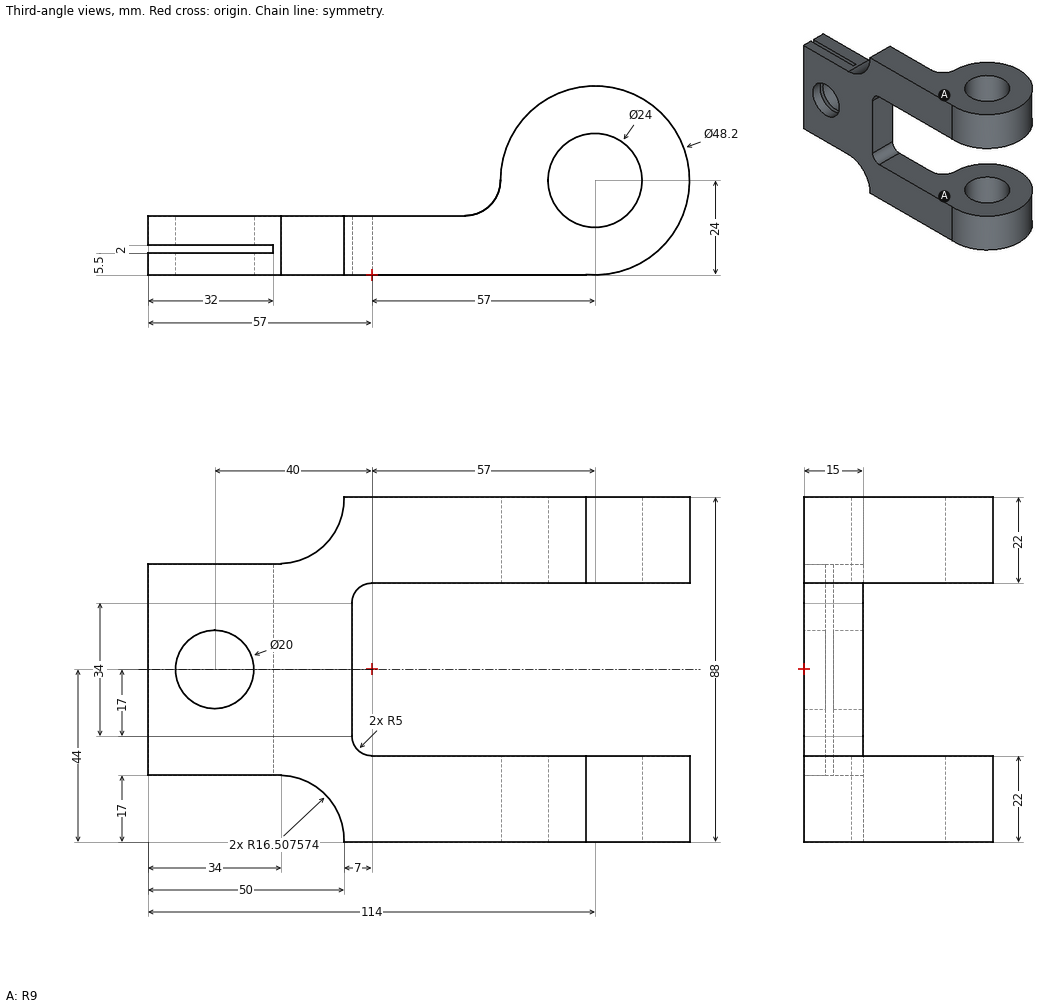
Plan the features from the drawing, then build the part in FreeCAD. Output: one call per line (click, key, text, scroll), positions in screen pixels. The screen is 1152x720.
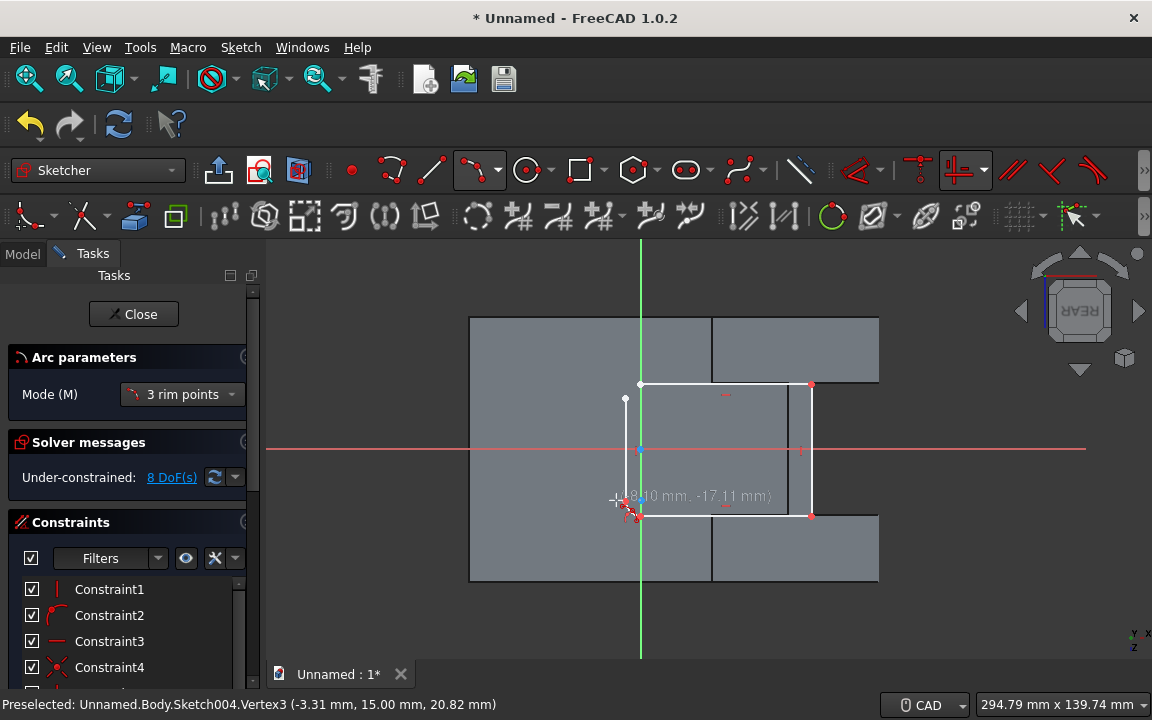
click(641, 384)
click(626, 399)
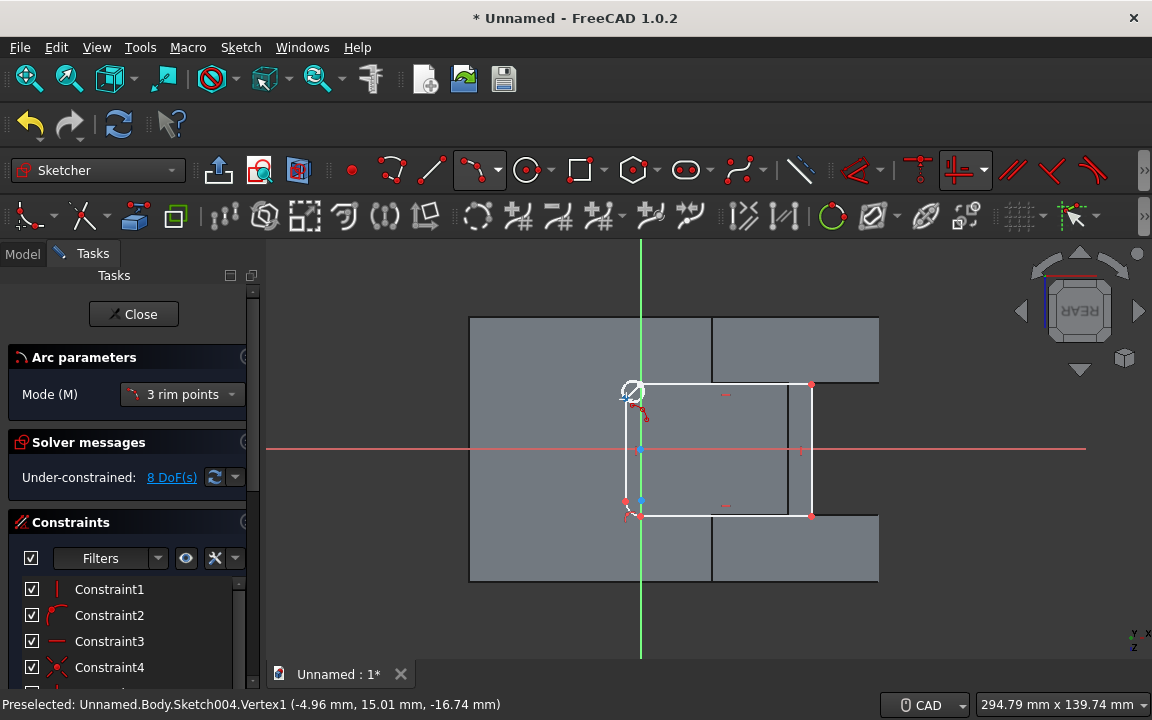
scroll(630, 388, up, 7)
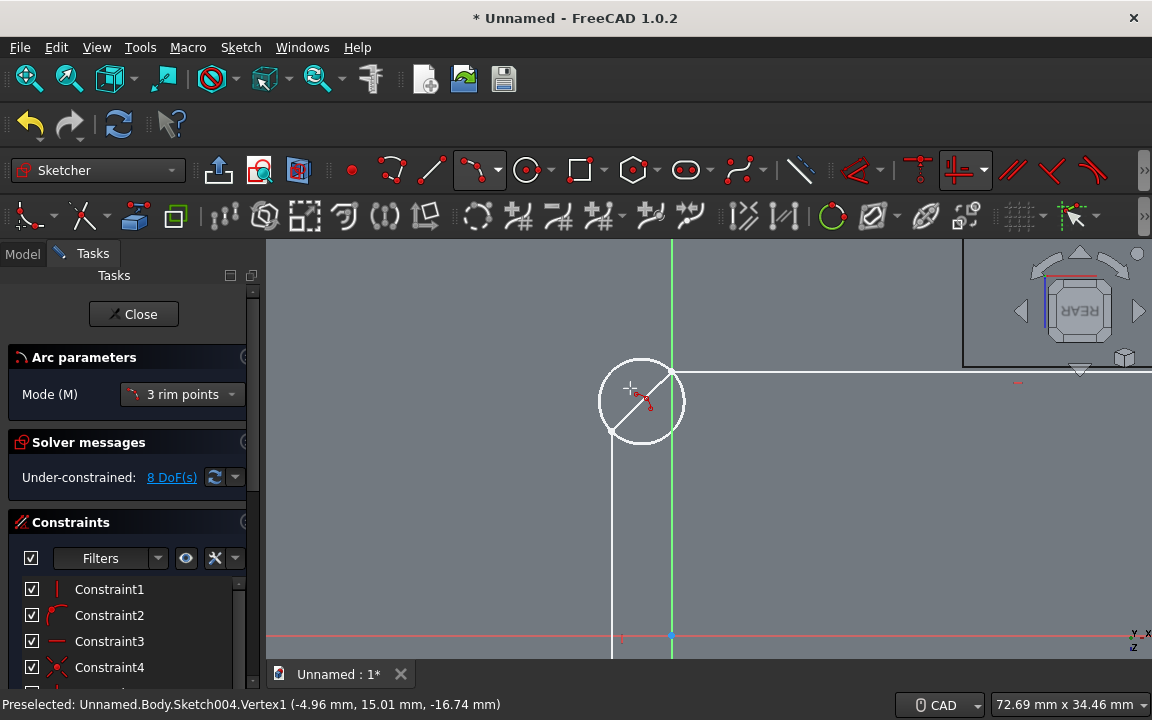
click(629, 385)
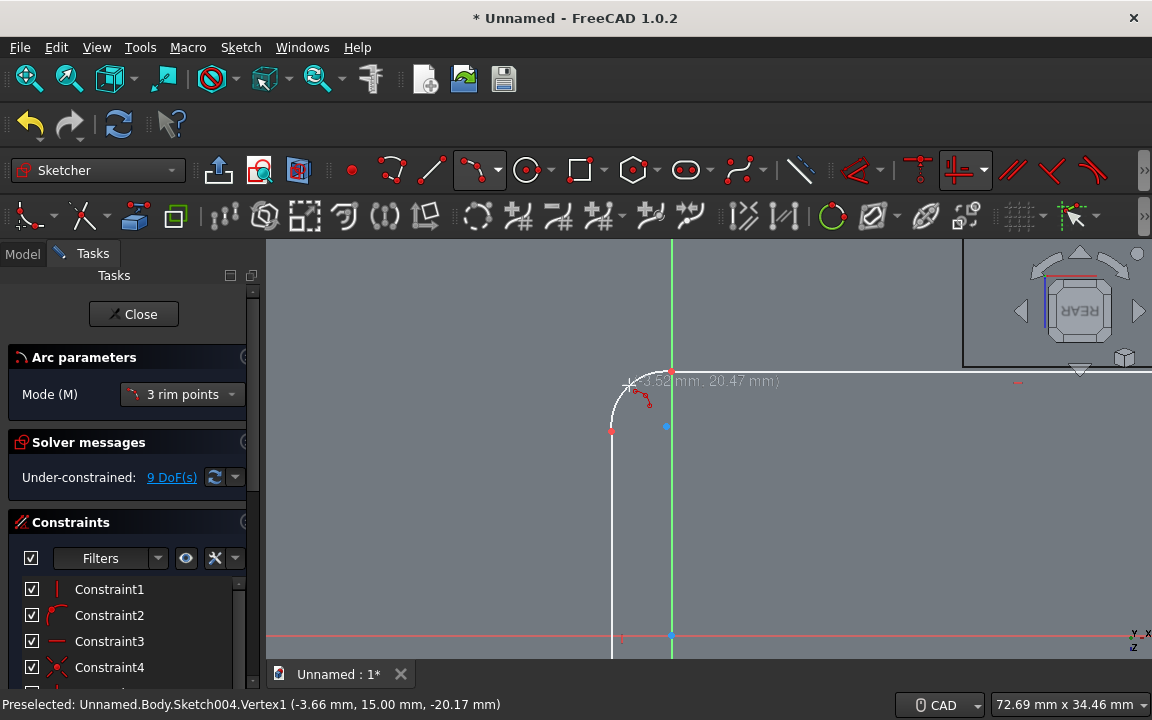
click(392, 170)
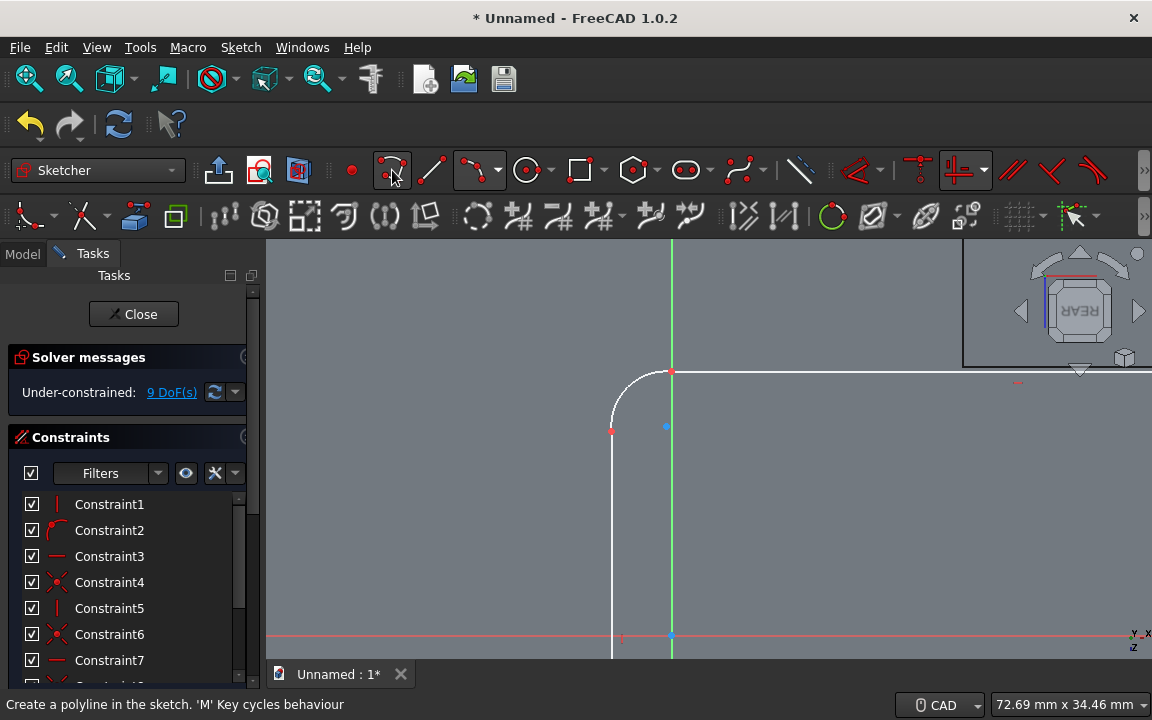
scroll(630, 388, down, 7)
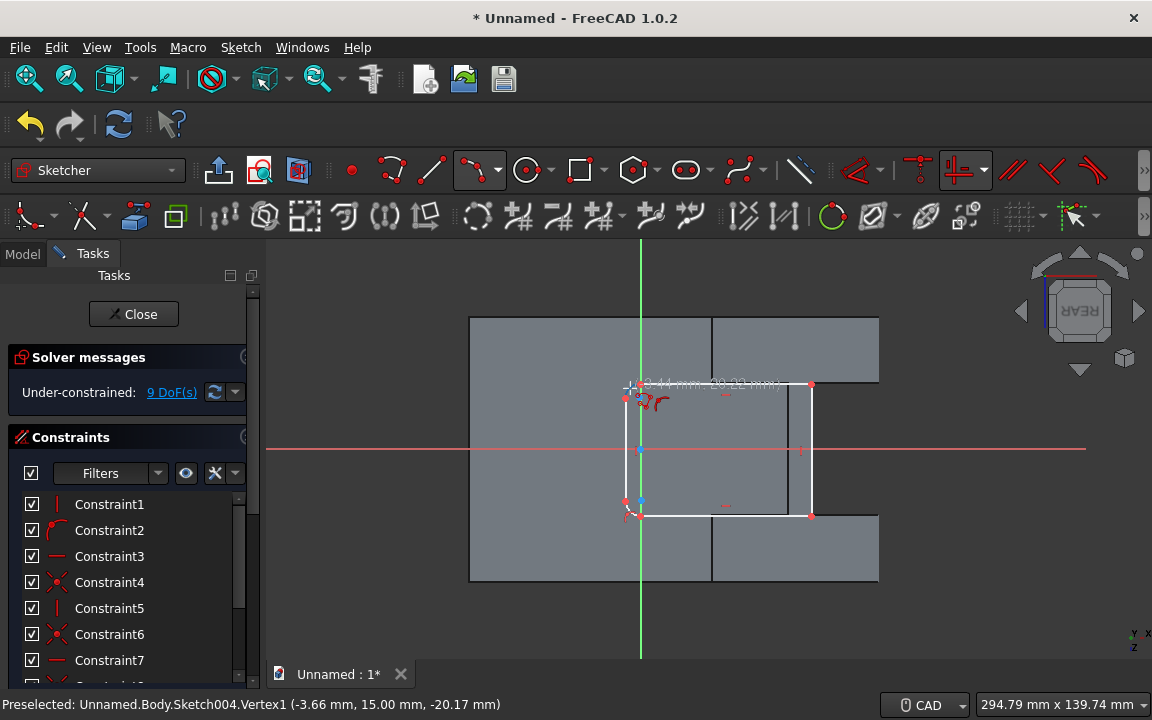
click(620, 317)
click(469, 317)
click(469, 368)
click(572, 368)
right_click(572, 368)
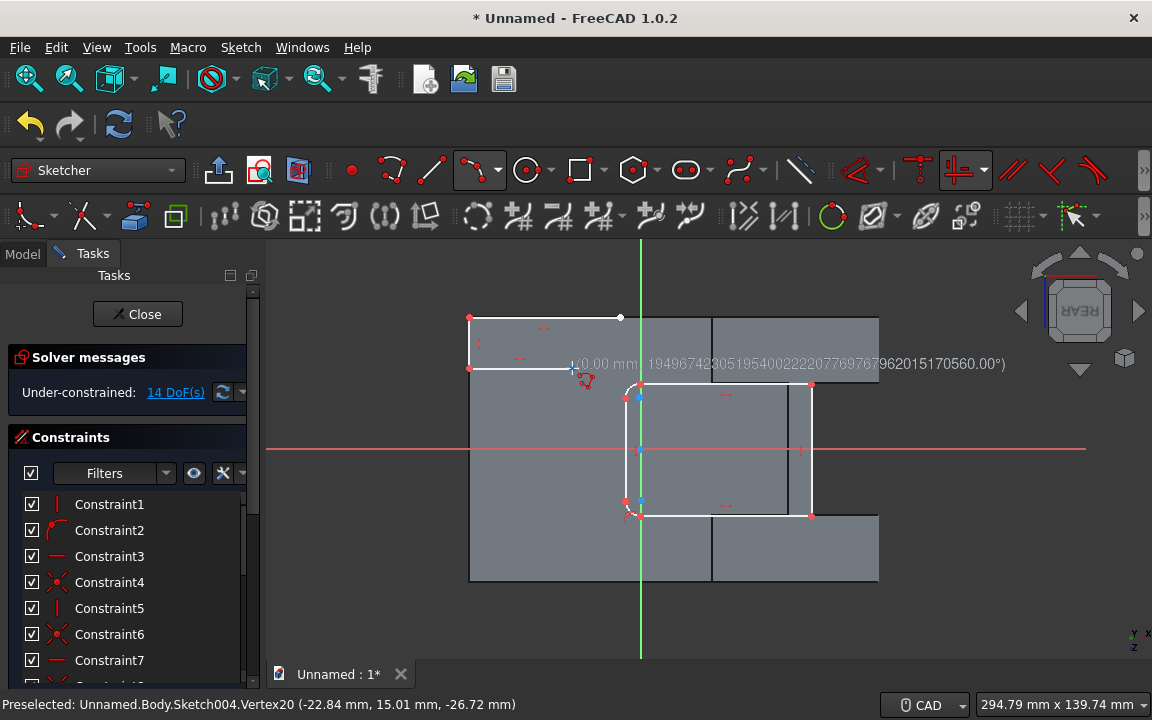
key(g)
key(3)
key(a)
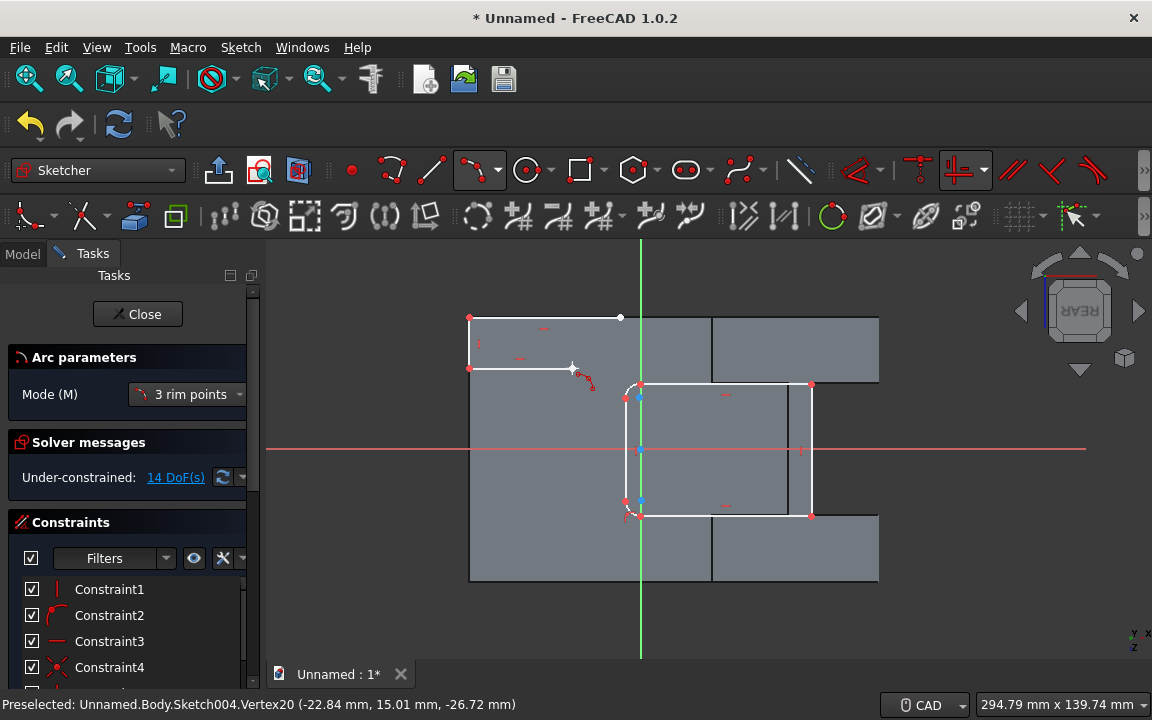
click(572, 369)
click(620, 318)
click(606, 353)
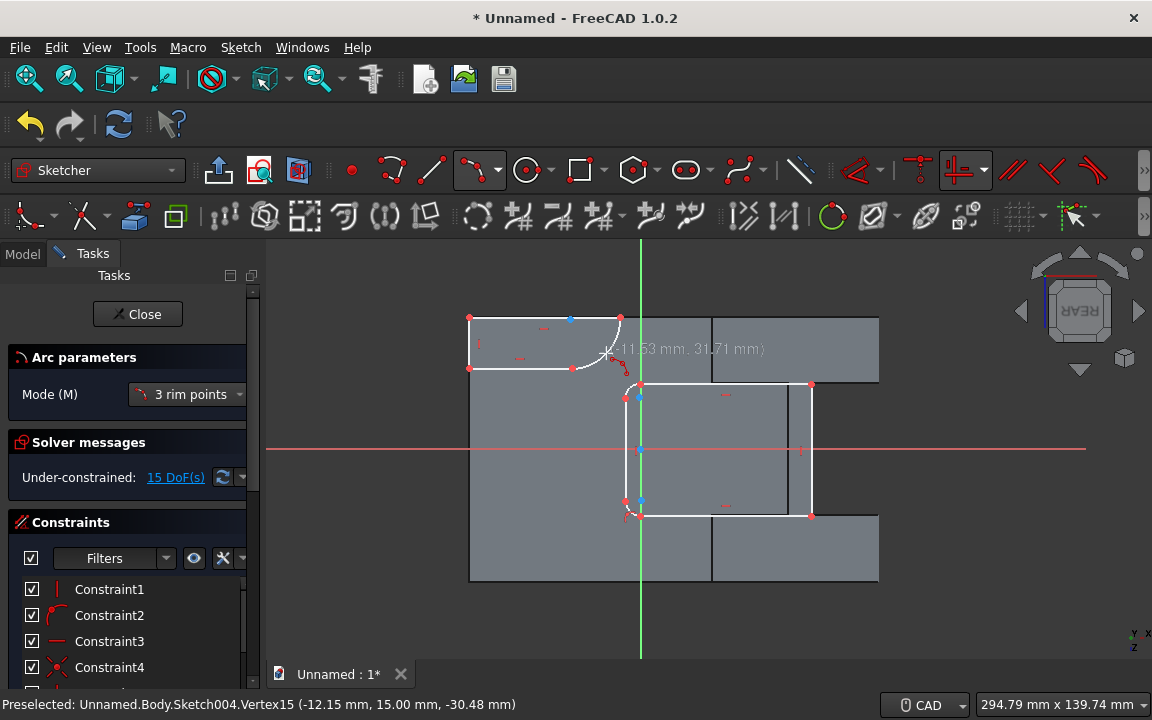
click(392, 170)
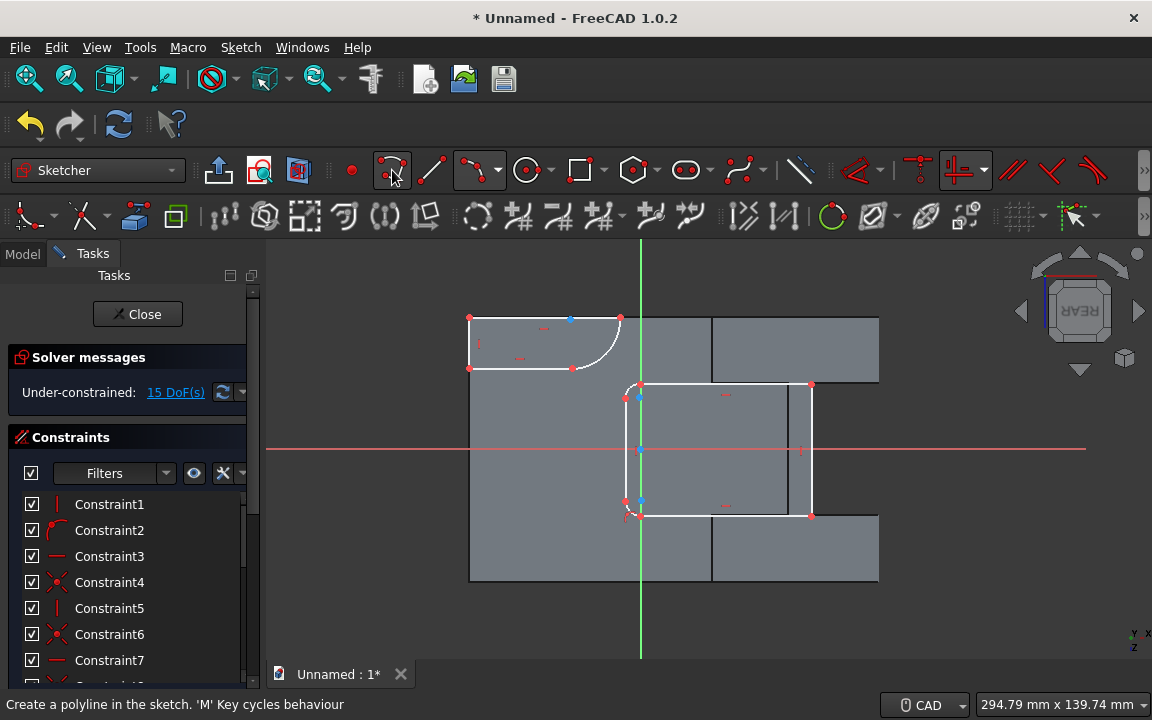
click(572, 530)
click(469, 530)
click(469, 582)
click(620, 582)
right_click(620, 582)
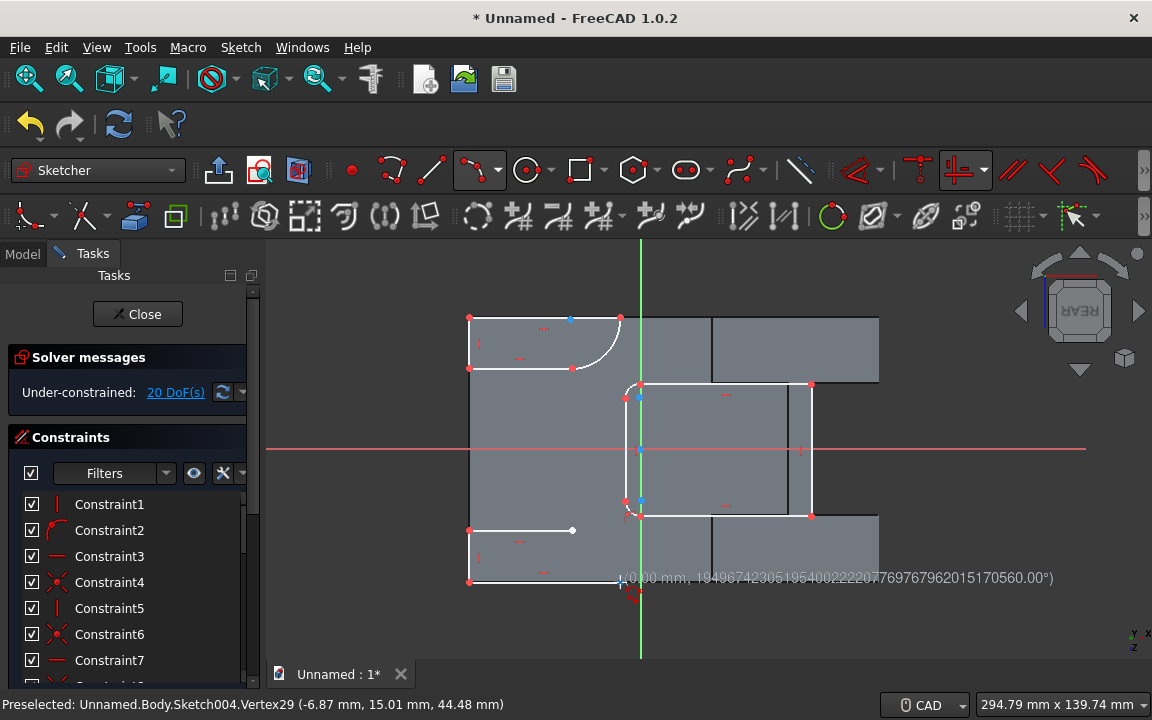
key(g)
key(3)
key(a)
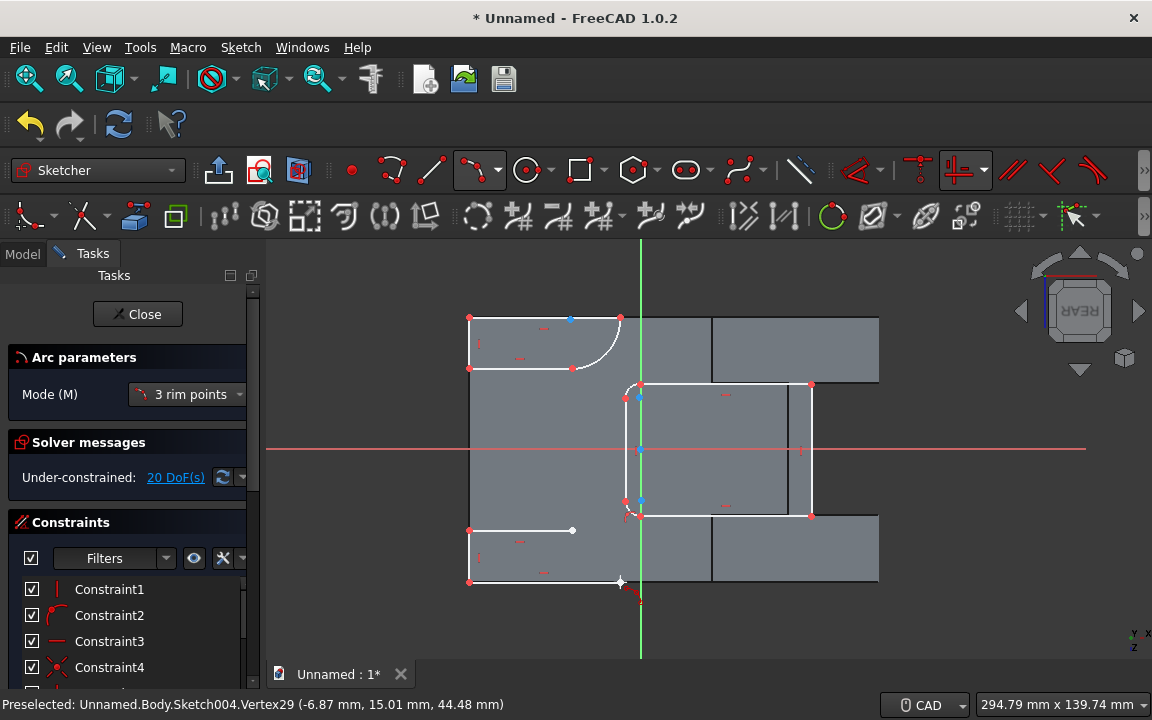
click(620, 583)
click(572, 531)
click(606, 546)